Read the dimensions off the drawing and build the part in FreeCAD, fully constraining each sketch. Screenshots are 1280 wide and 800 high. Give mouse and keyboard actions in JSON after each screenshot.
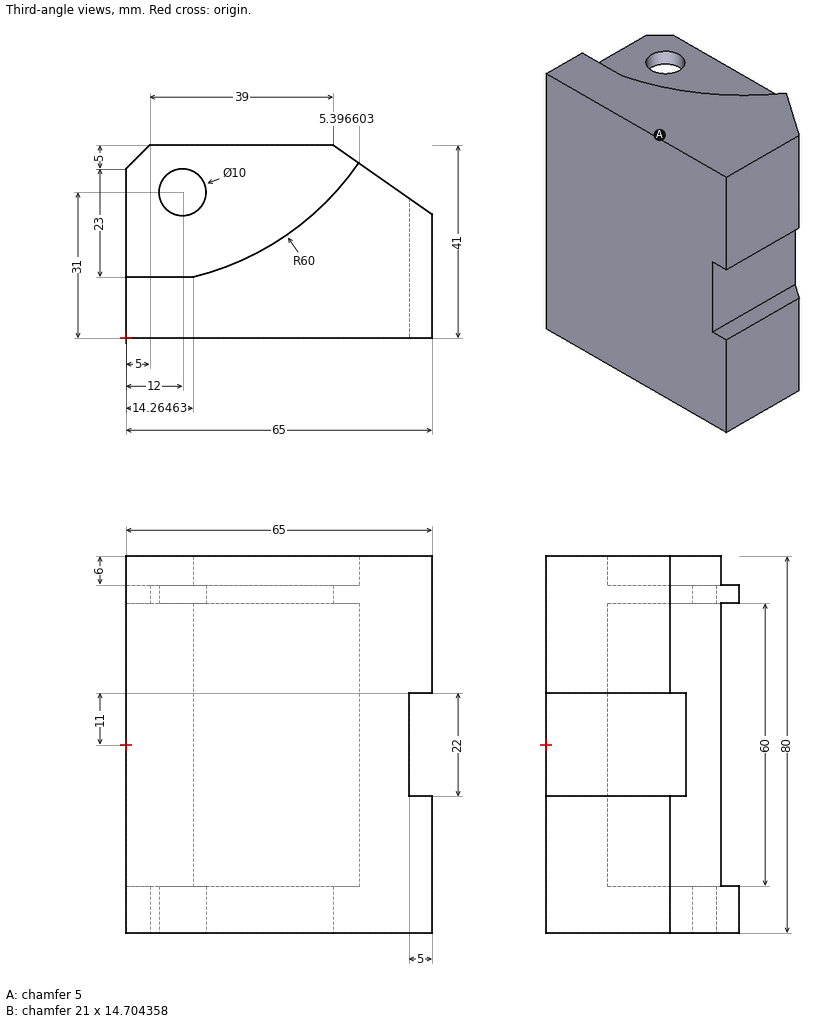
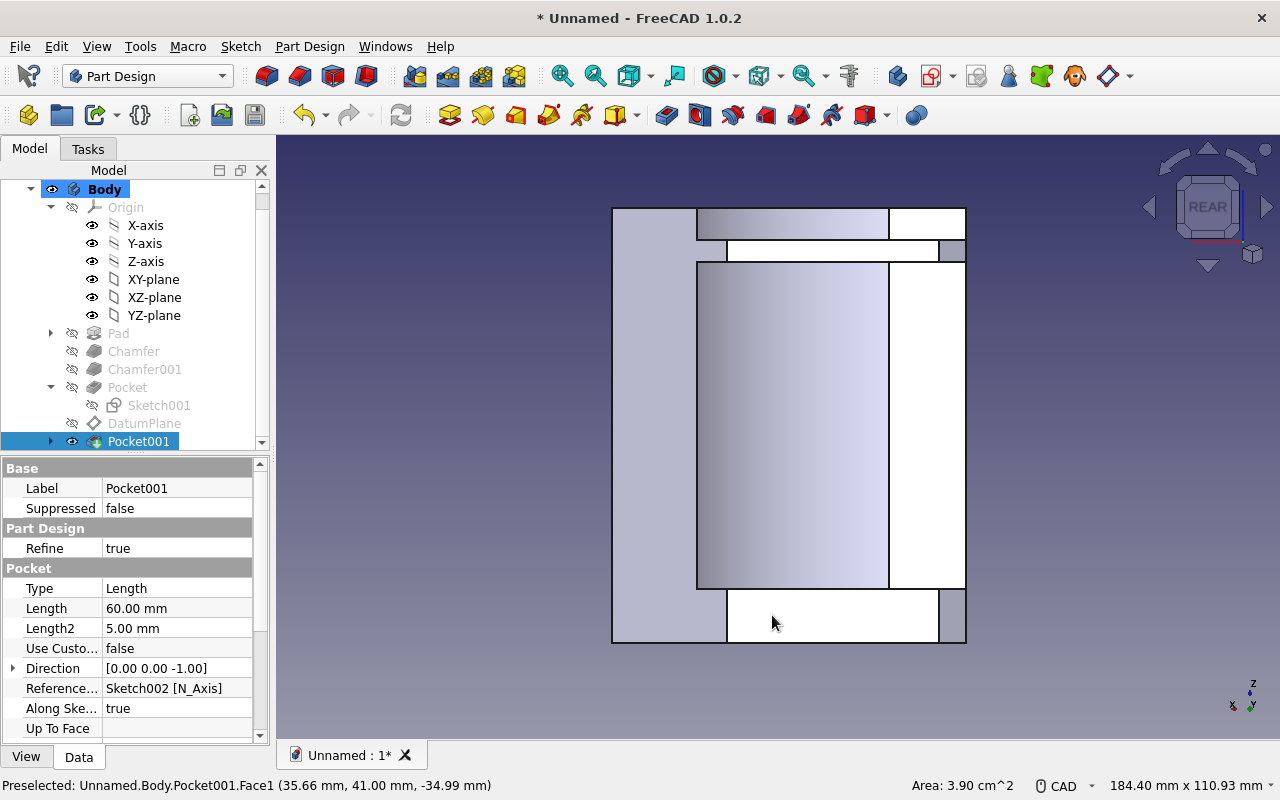
{"action": "left_click", "coordinate": [930, 76]}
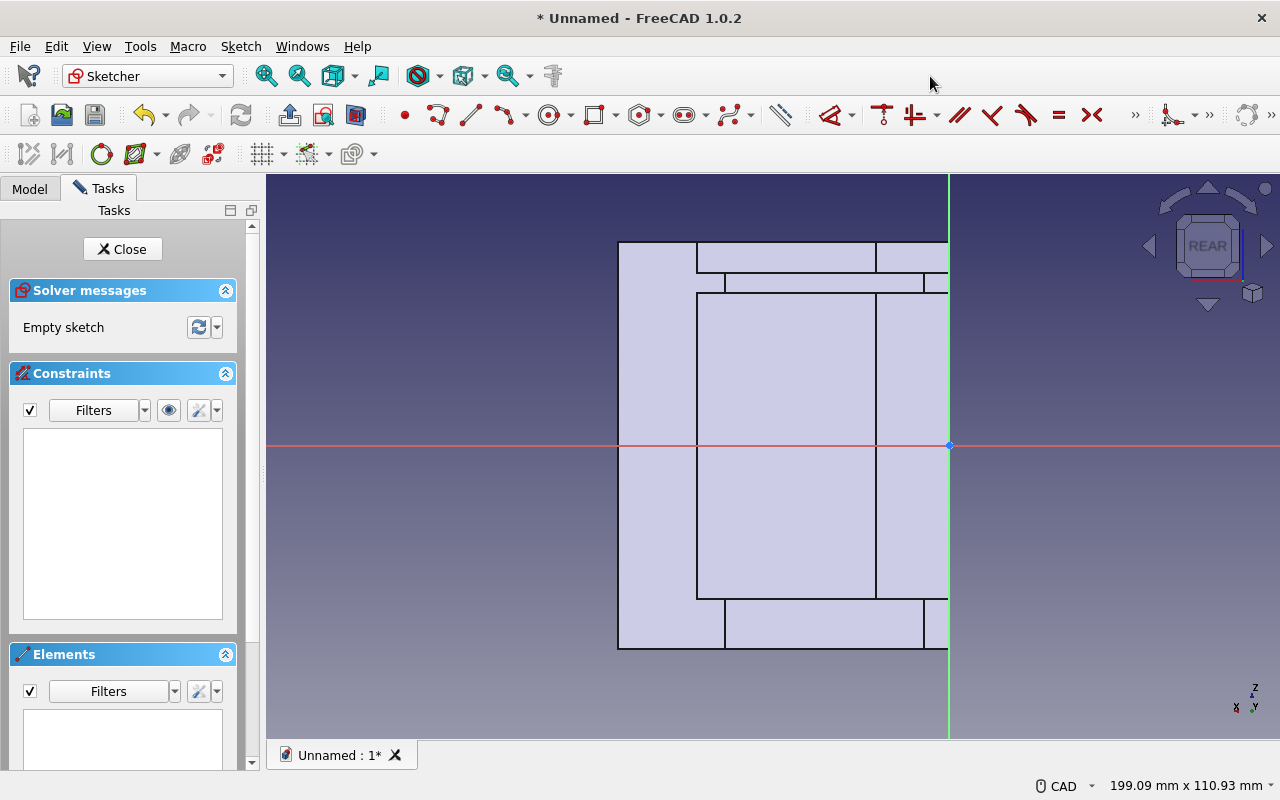
{"action": "scroll", "coordinate": [599, 441], "scroll_direction": "up", "scroll_amount": 6}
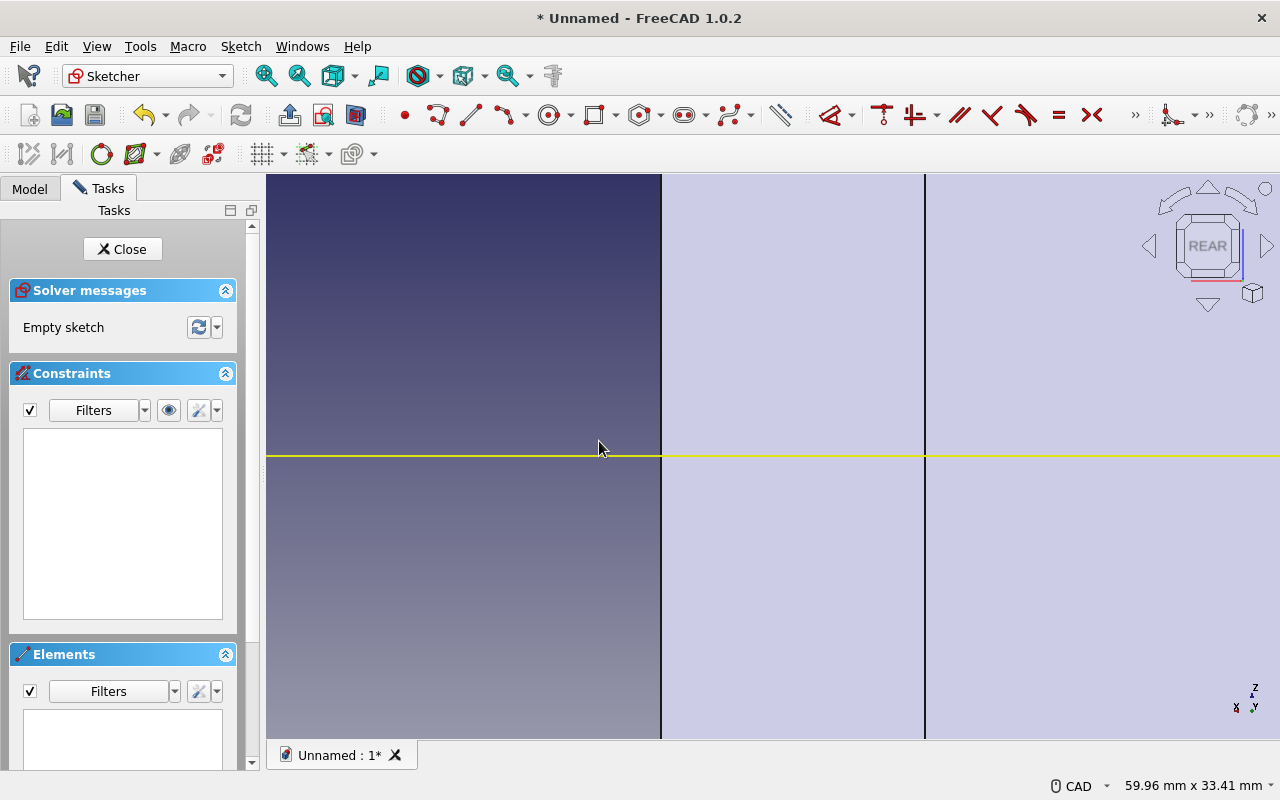
{"action": "key", "text": "g r"}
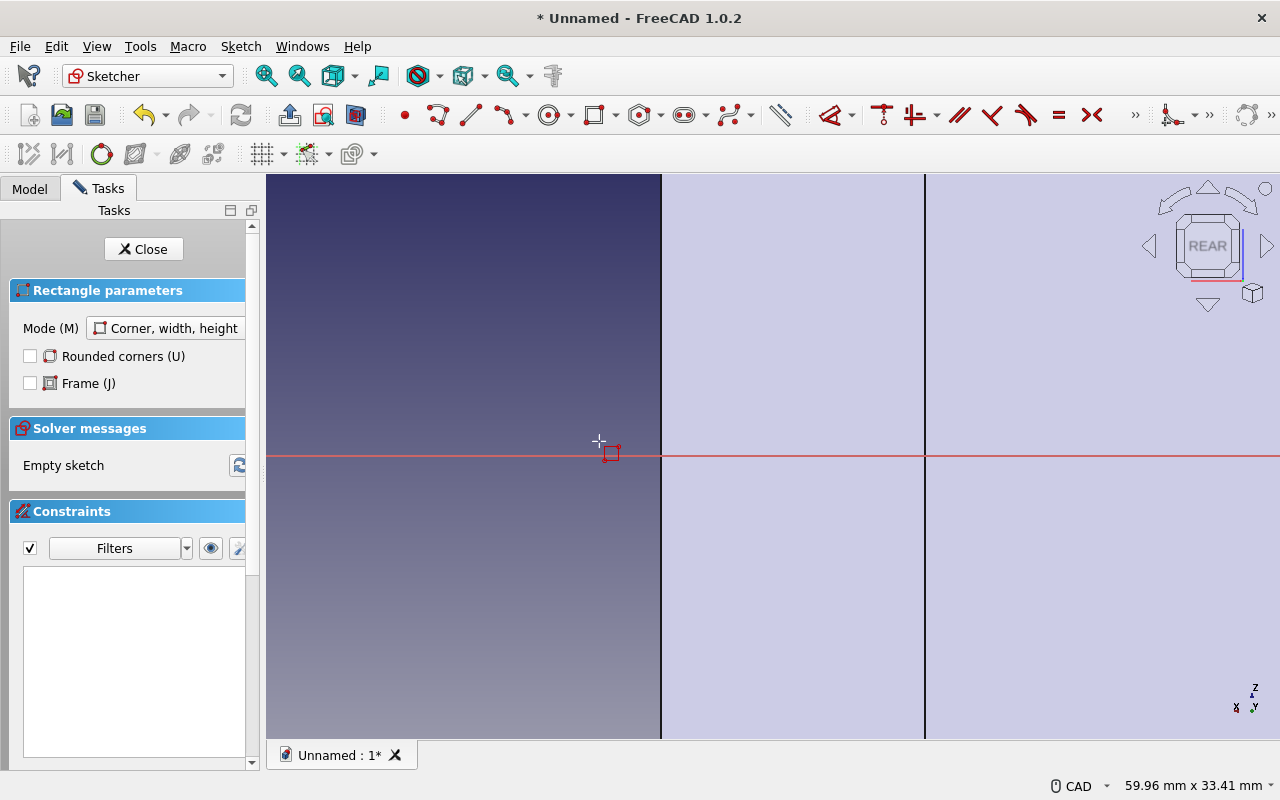
{"action": "left_click", "coordinate": [661, 270]}
{"action": "left_click", "coordinate": [746, 642]}
{"action": "key", "text": "Escape"}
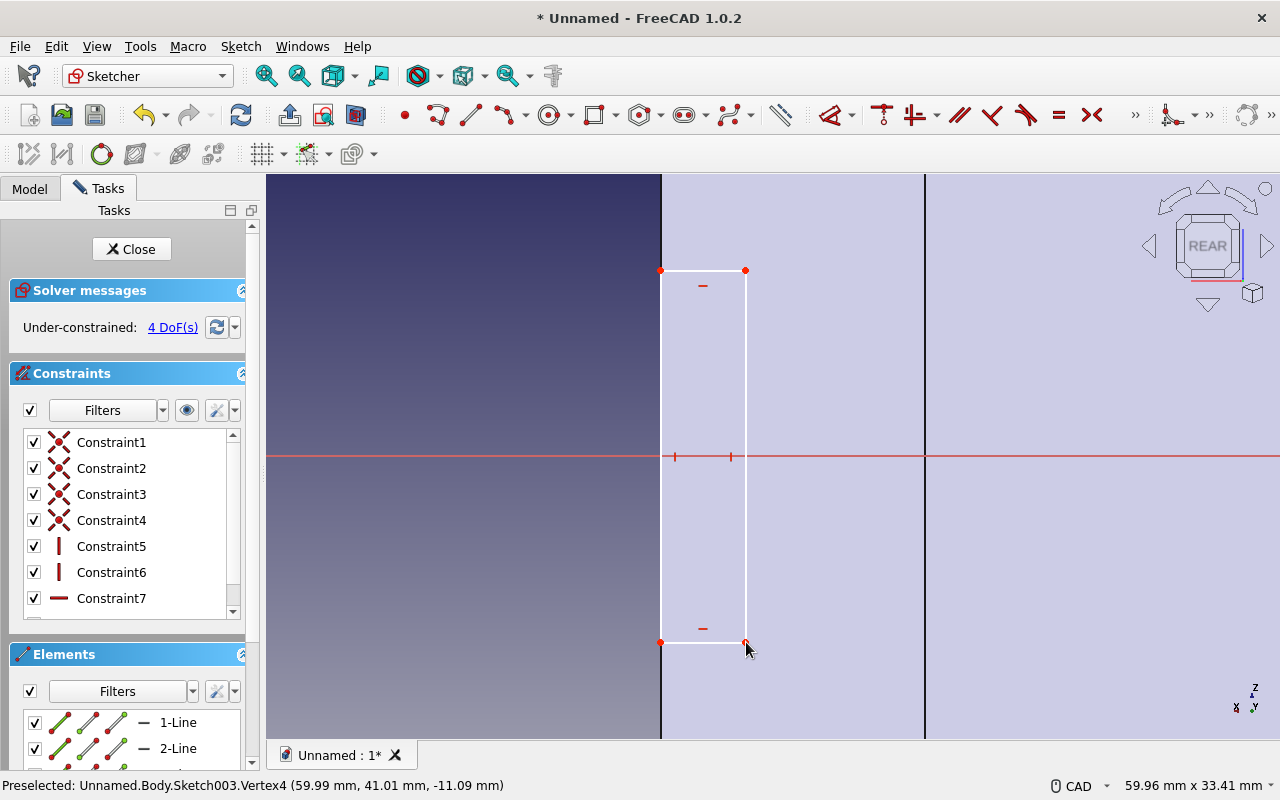
{"action": "key", "text": "d"}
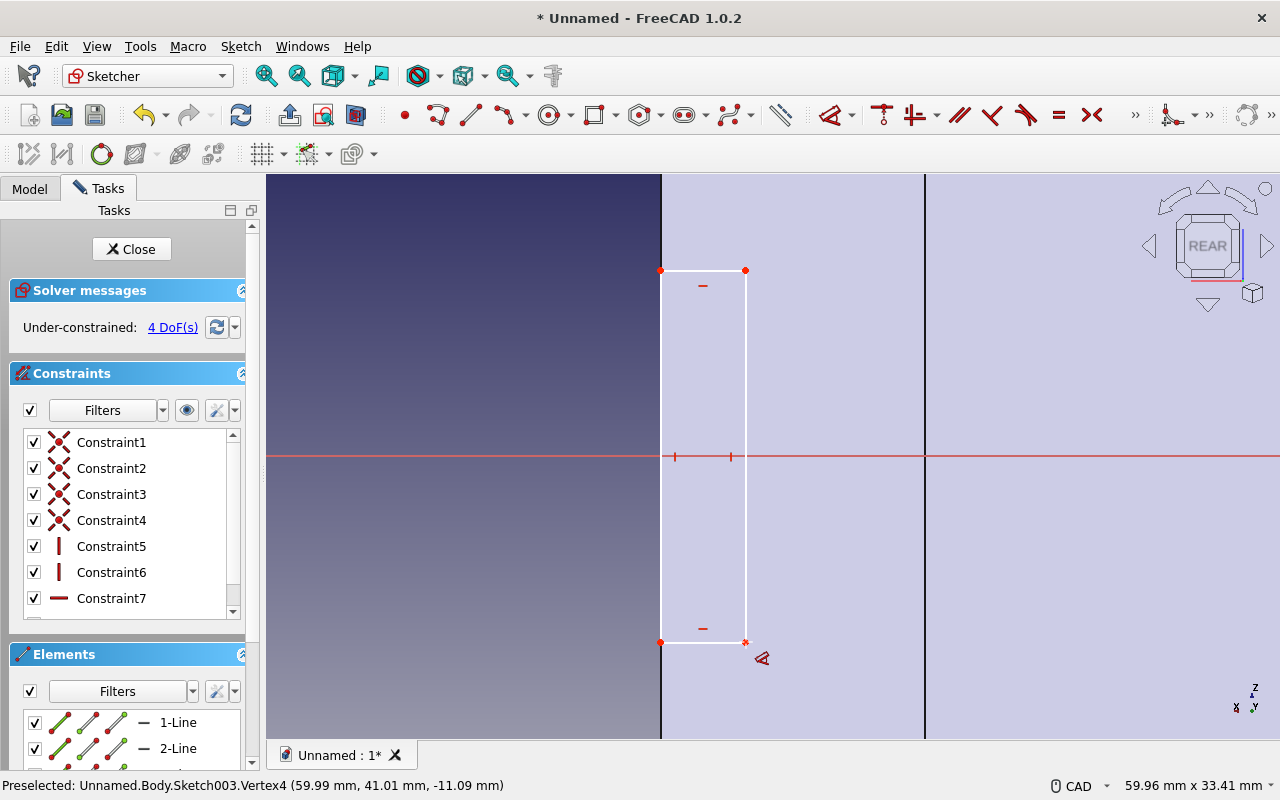
{"action": "left_click", "coordinate": [686, 643]}
{"action": "left_click", "coordinate": [703, 677]}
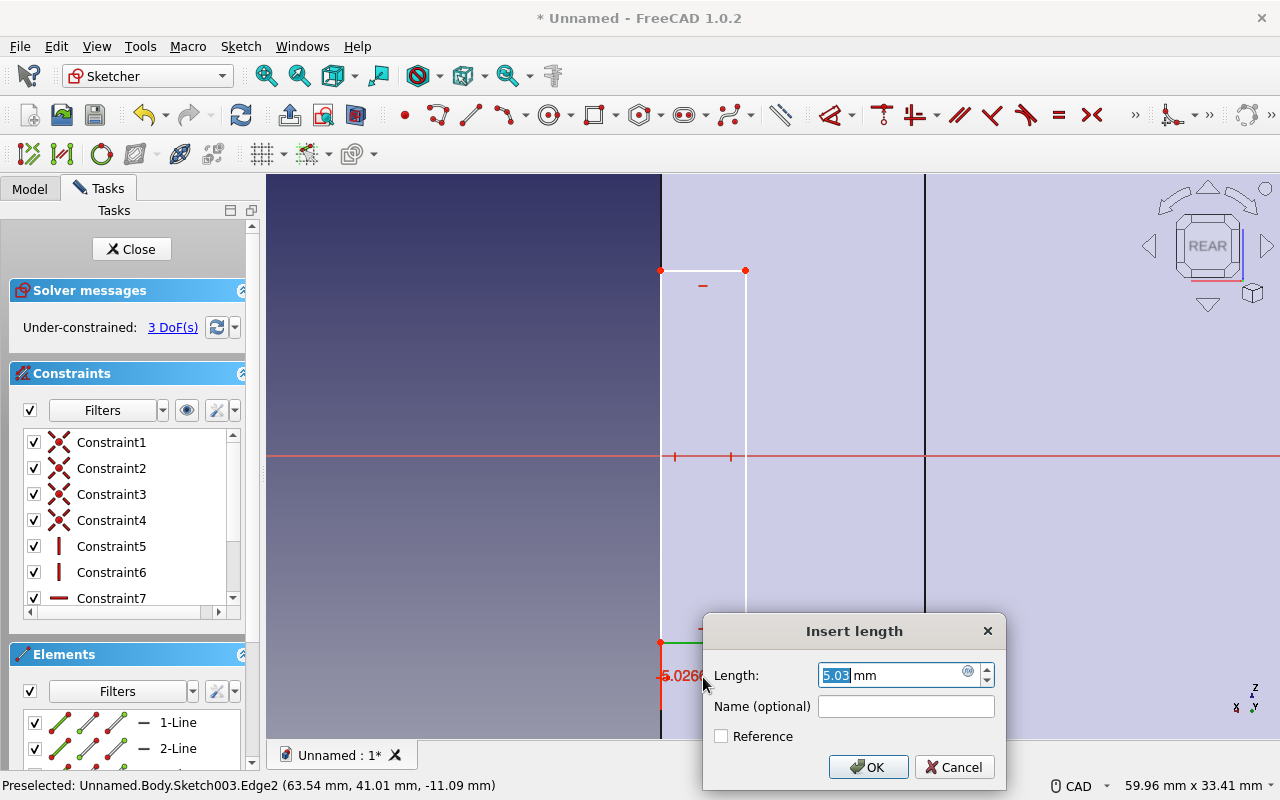
{"action": "type", "text": "5"}
{"action": "key", "text": "Return"}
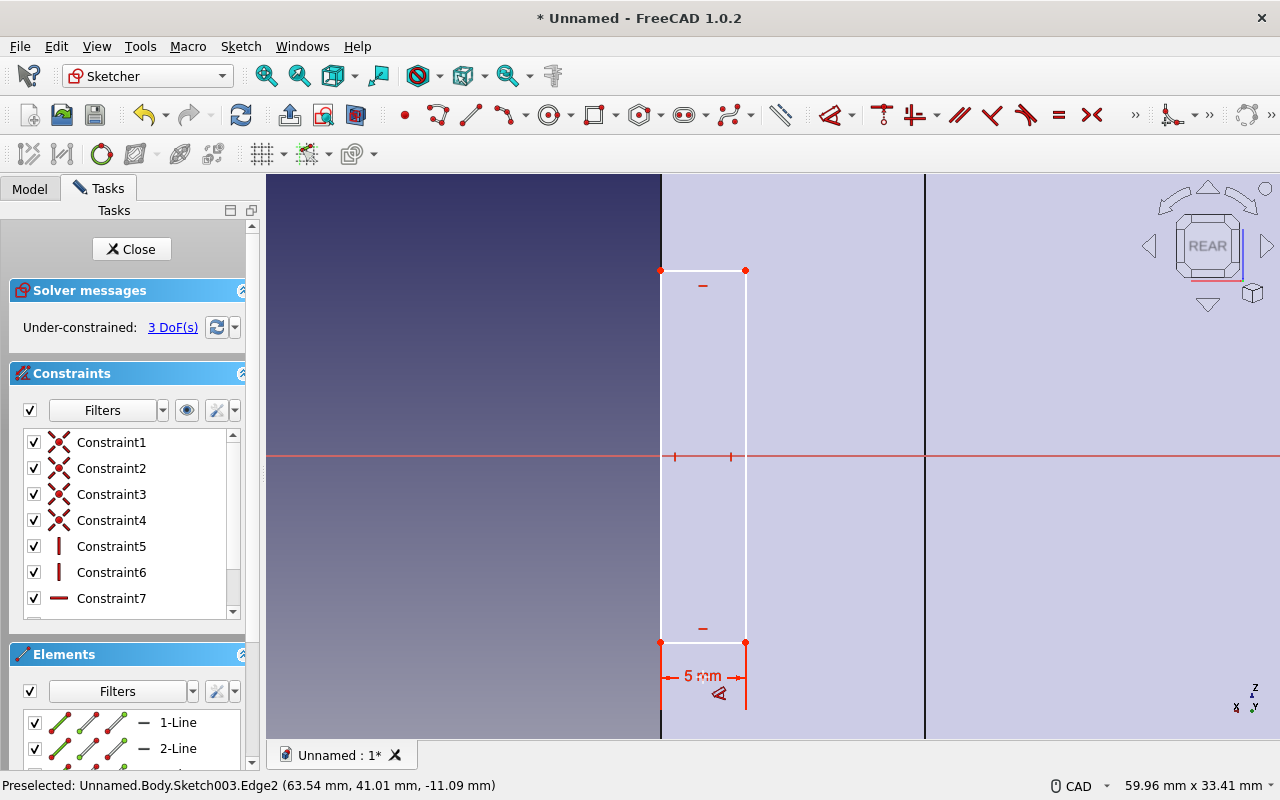
{"action": "left_click", "coordinate": [661, 383]}
{"action": "left_click", "coordinate": [627, 371]}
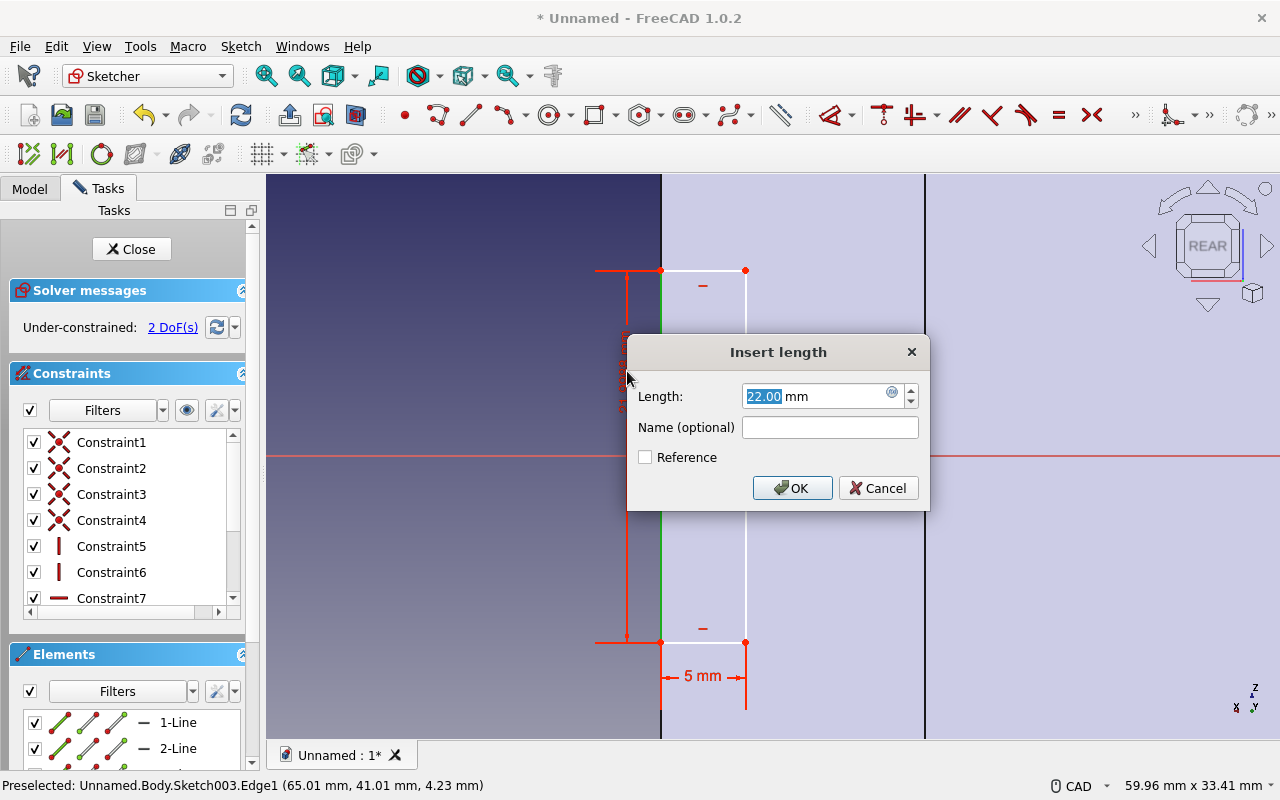
{"action": "type", "text": "22"}
{"action": "key", "text": "Return"}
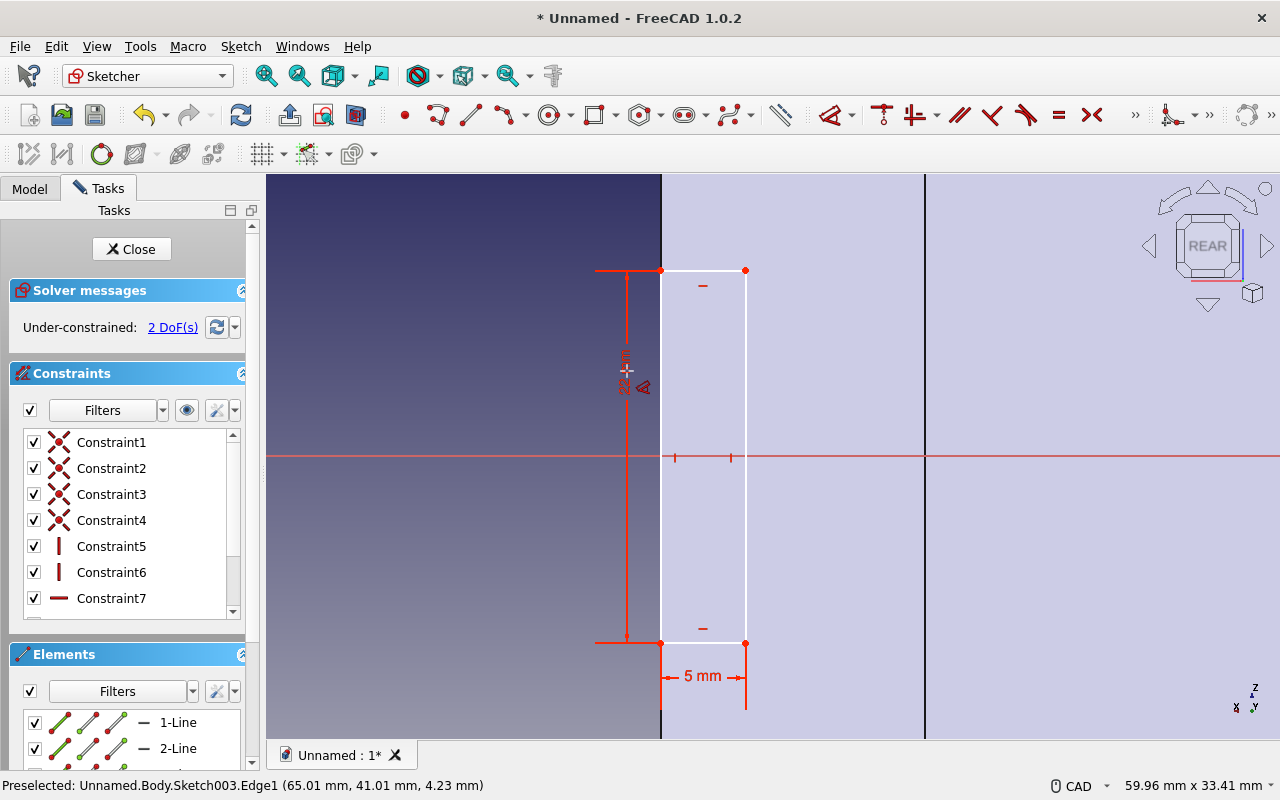
{"action": "left_click", "coordinate": [661, 271]}
{"action": "left_click", "coordinate": [888, 237]}